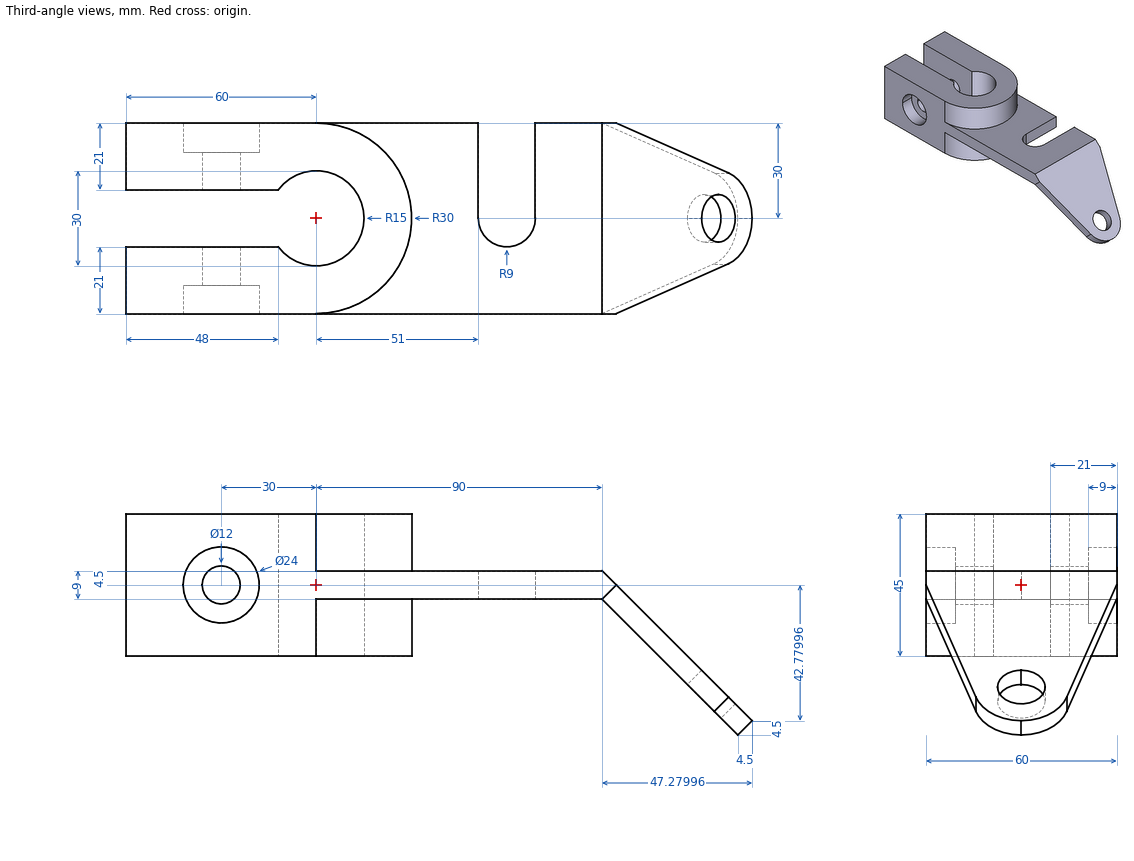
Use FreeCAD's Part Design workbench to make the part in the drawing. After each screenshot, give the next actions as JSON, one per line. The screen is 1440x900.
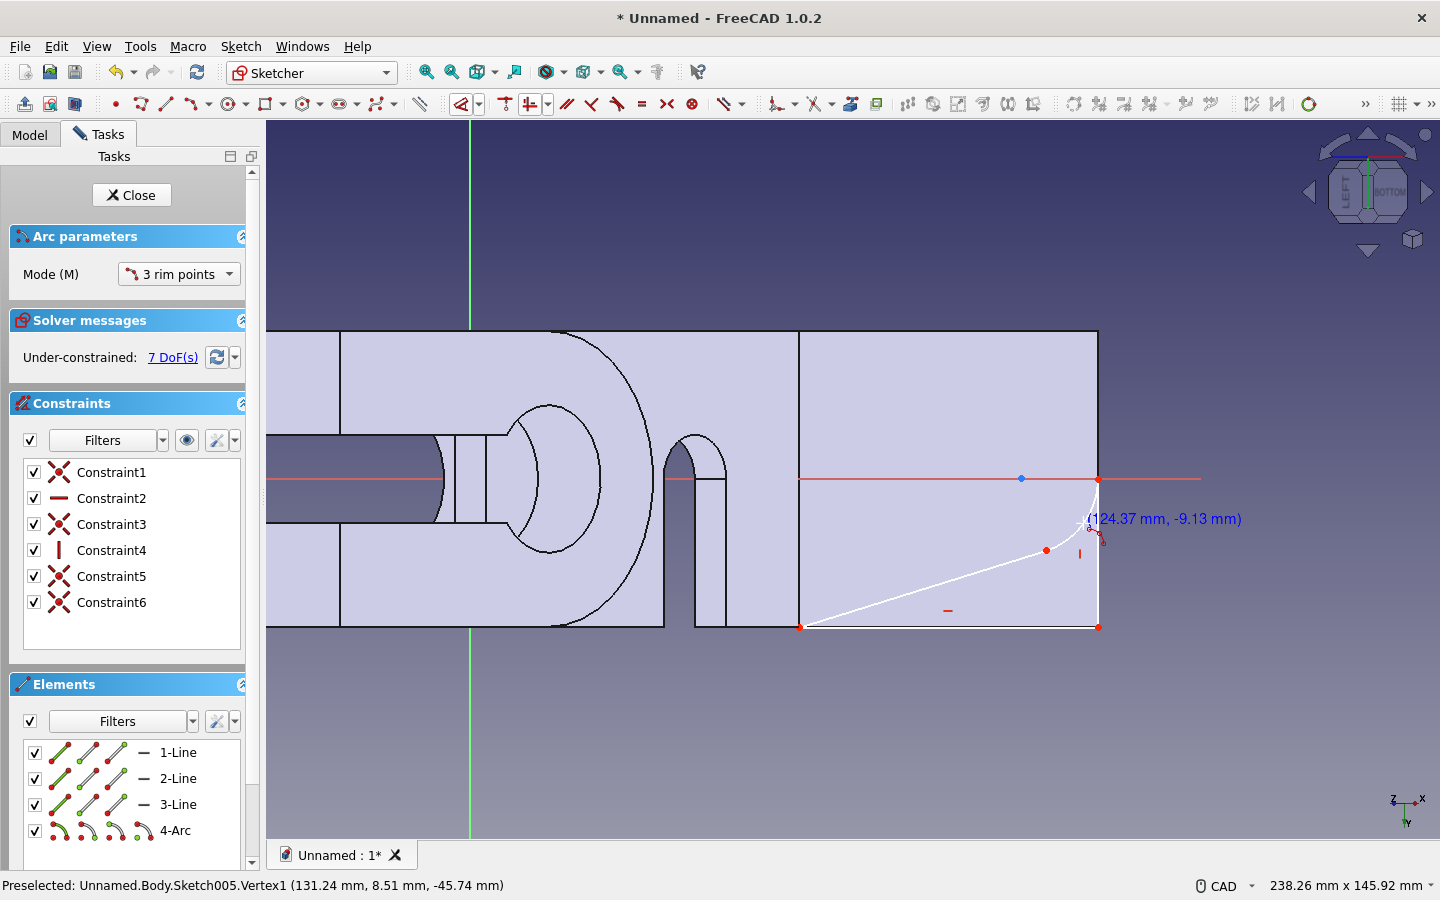
{"action": "left_click", "coordinate": [141, 104]}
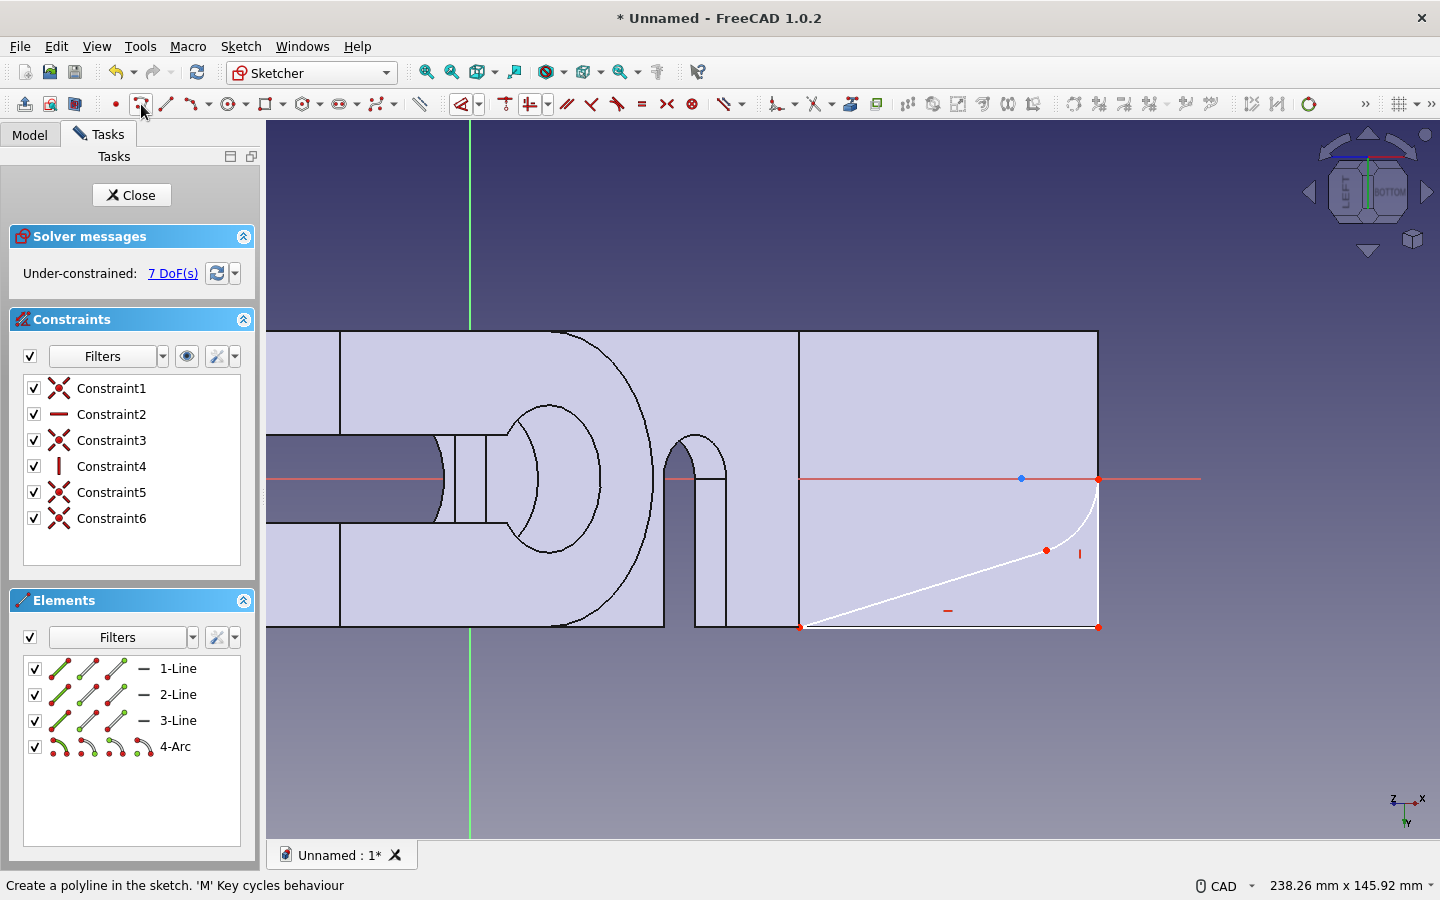
{"action": "left_click", "coordinate": [1098, 479]}
{"action": "left_click", "coordinate": [1098, 331]}
{"action": "left_click", "coordinate": [799, 331]}
{"action": "left_click", "coordinate": [1046, 408]}
{"action": "right_click", "coordinate": [1046, 408]}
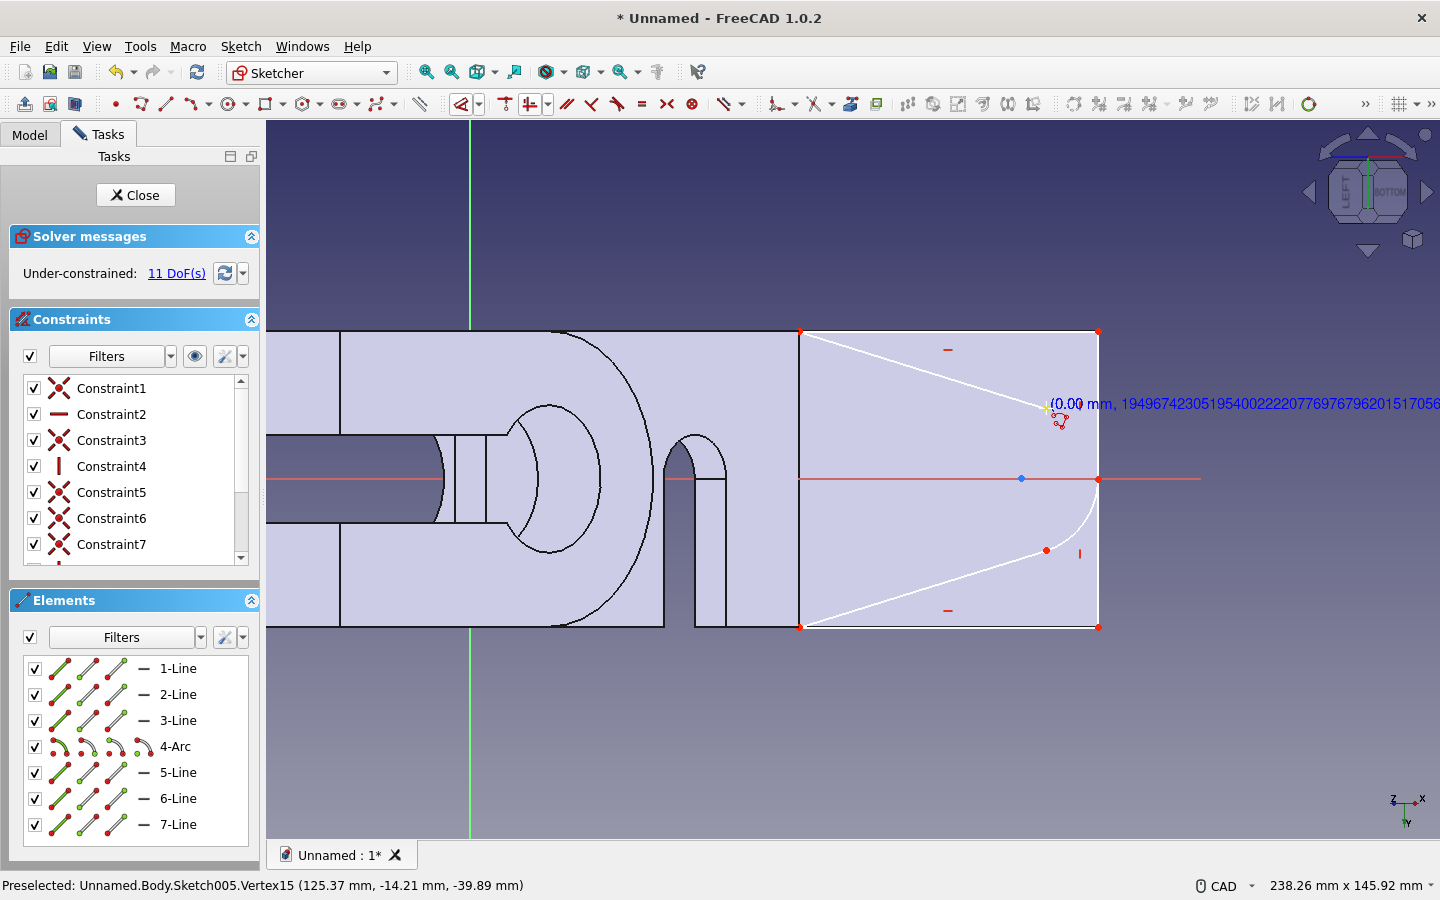
{"action": "key", "text": "g 3 a"}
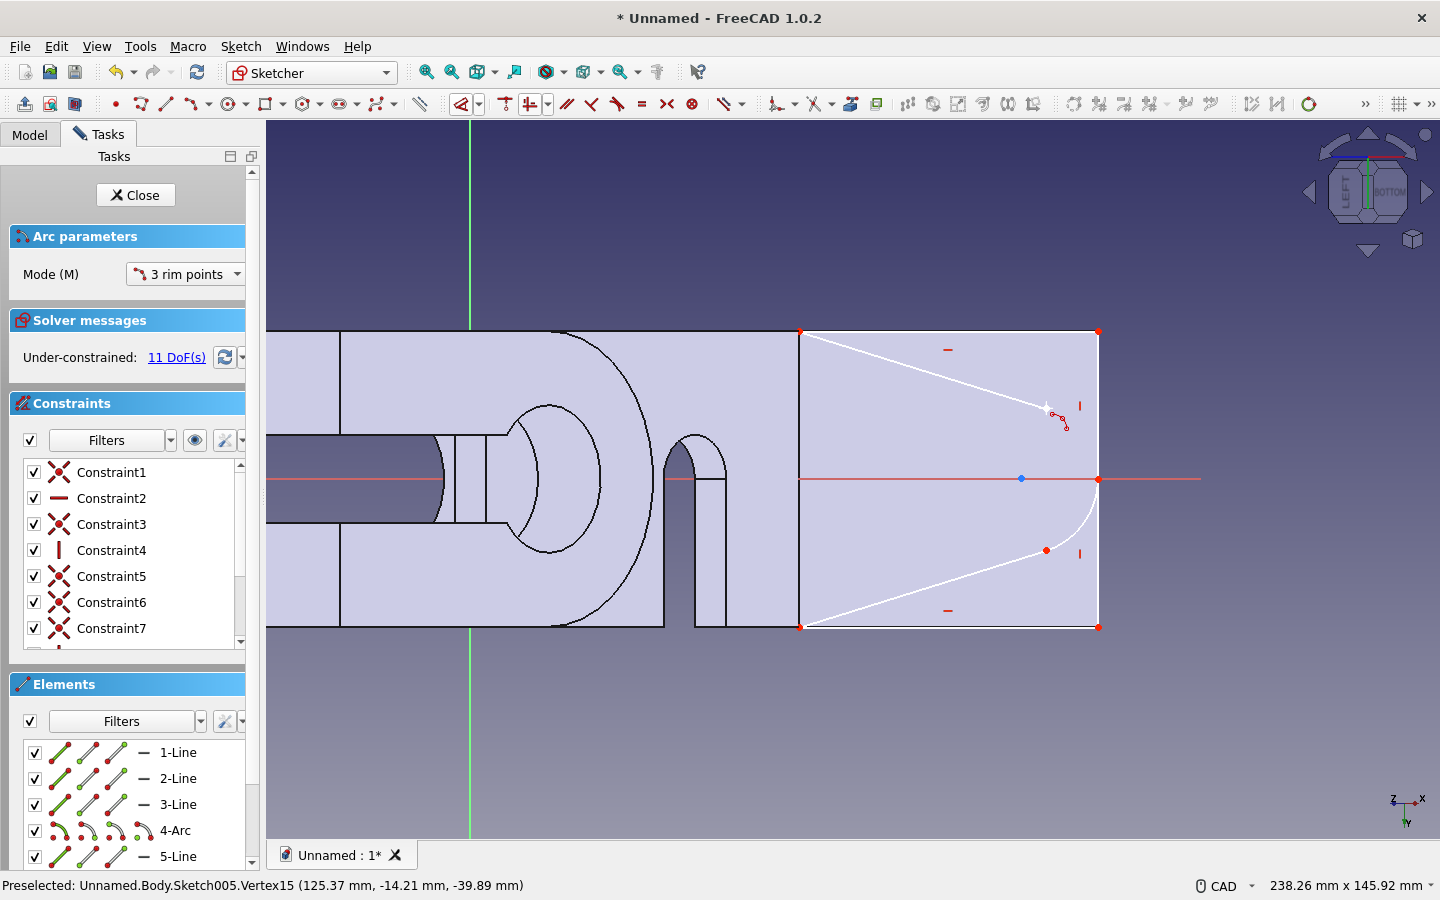
{"action": "left_click", "coordinate": [1046, 409]}
{"action": "left_click", "coordinate": [1098, 479]}
{"action": "left_click", "coordinate": [1083, 435]}
{"action": "key", "text": "Escape"}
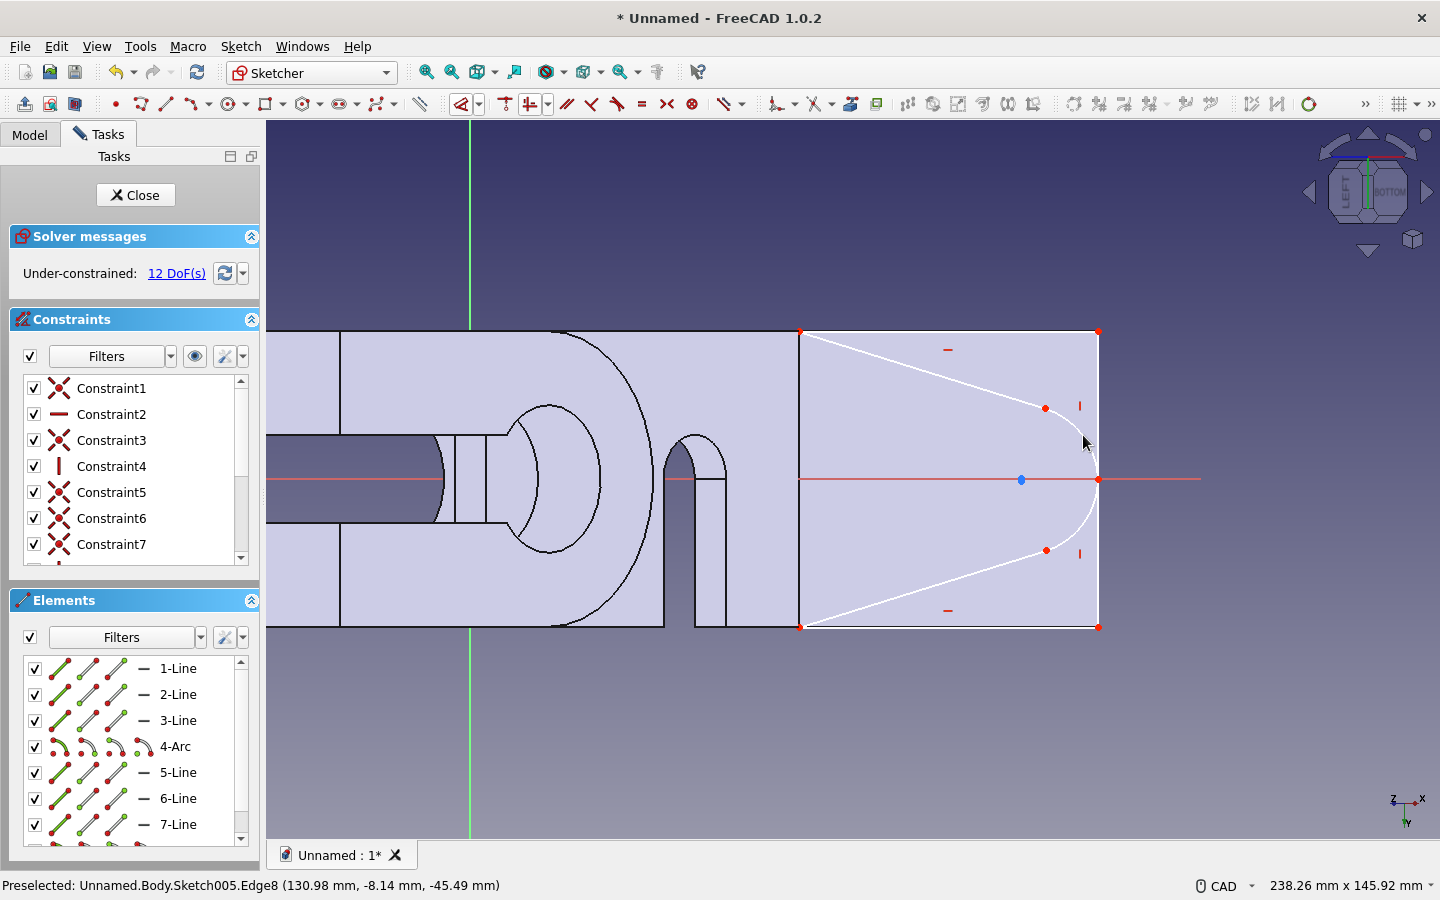
{"action": "left_click", "coordinate": [972, 574]}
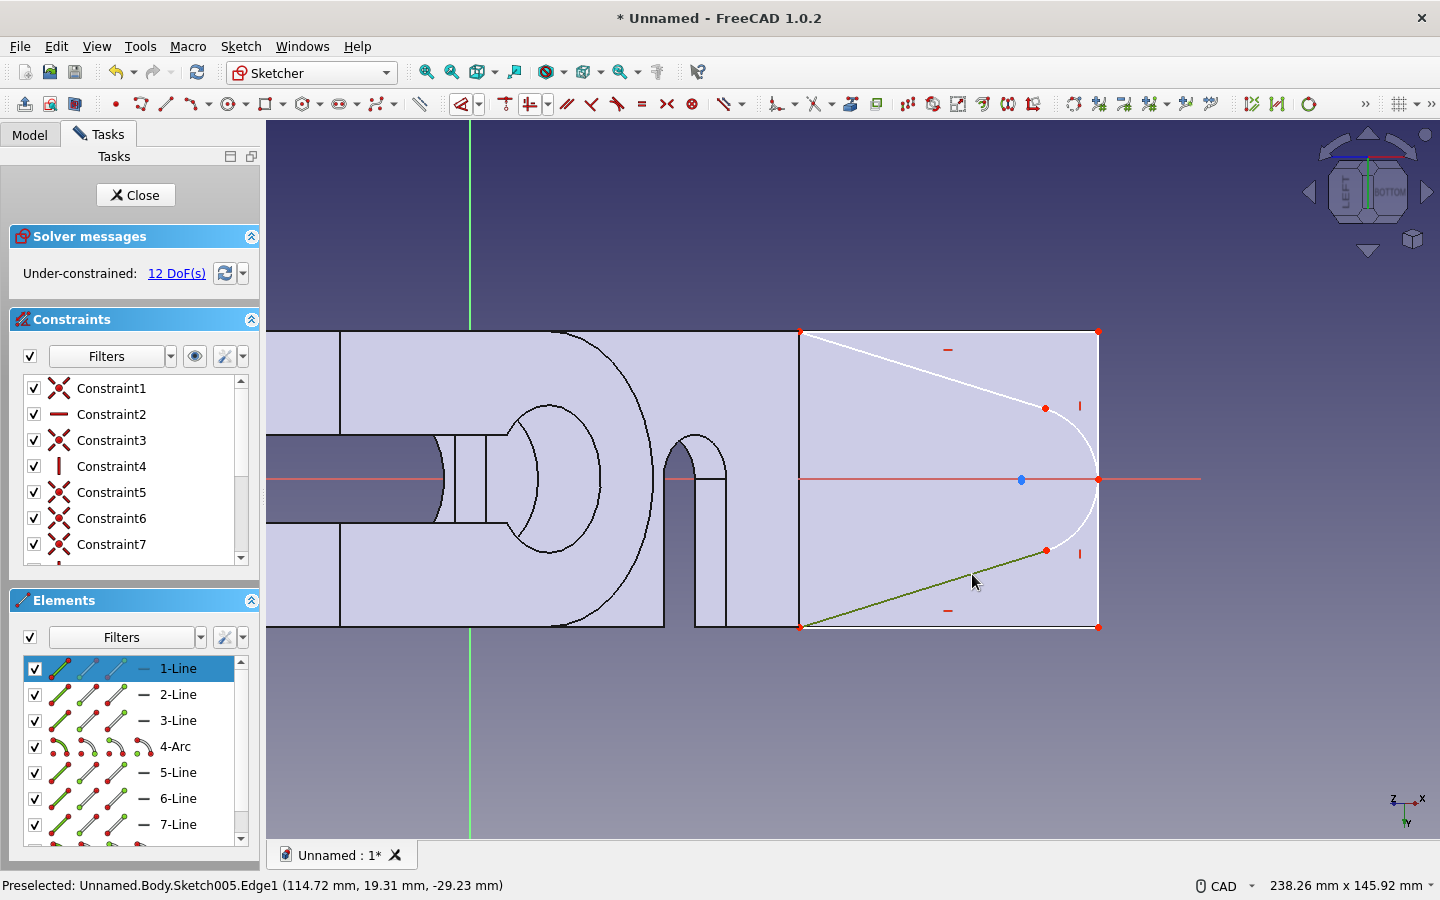
{"action": "left_click", "coordinate": [1071, 537]}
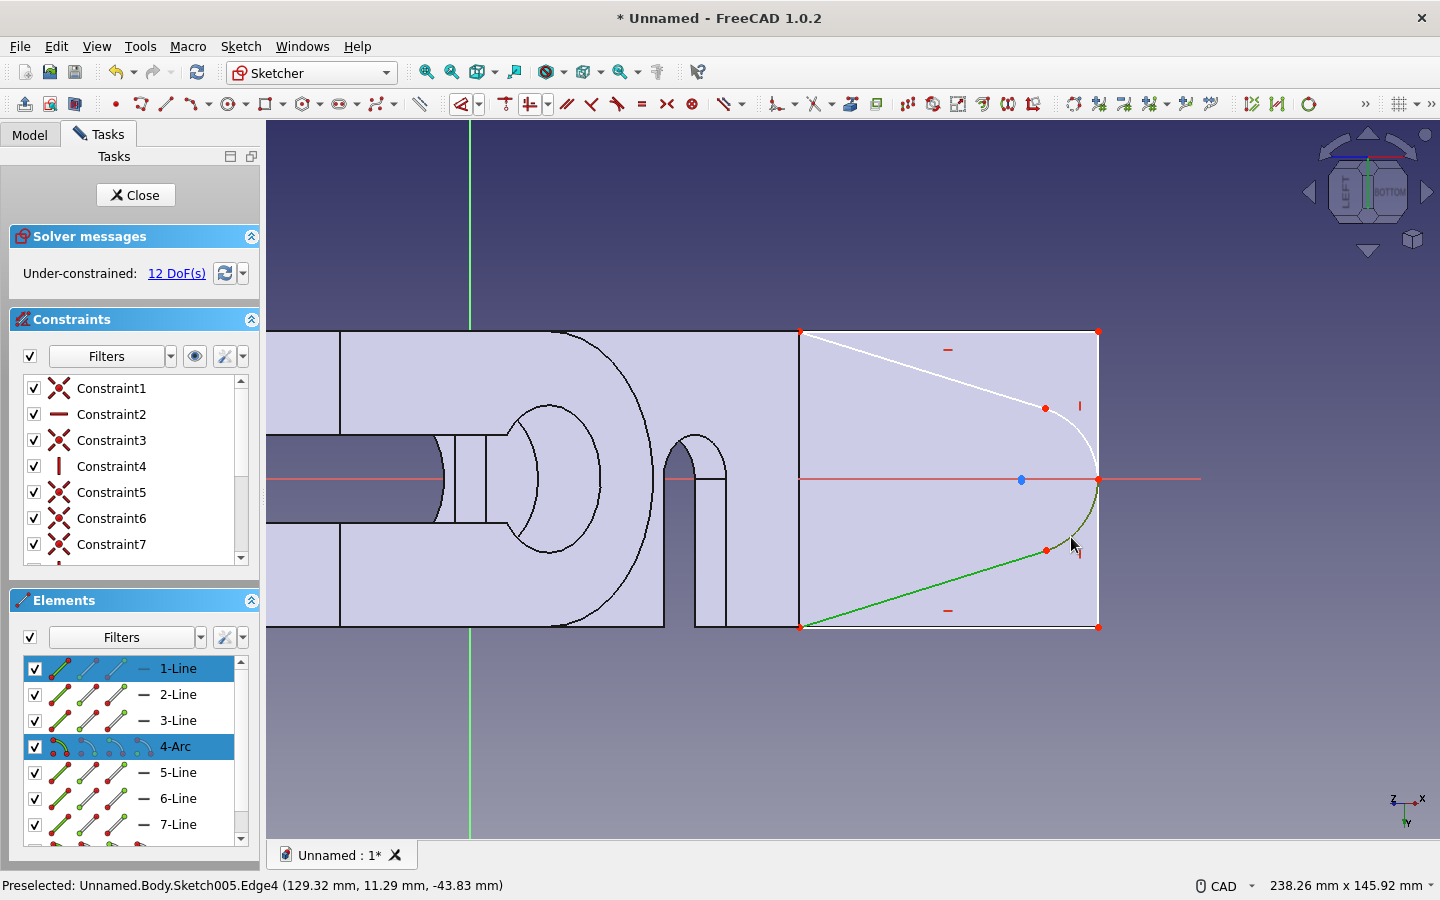
{"action": "left_click", "coordinate": [617, 104]}